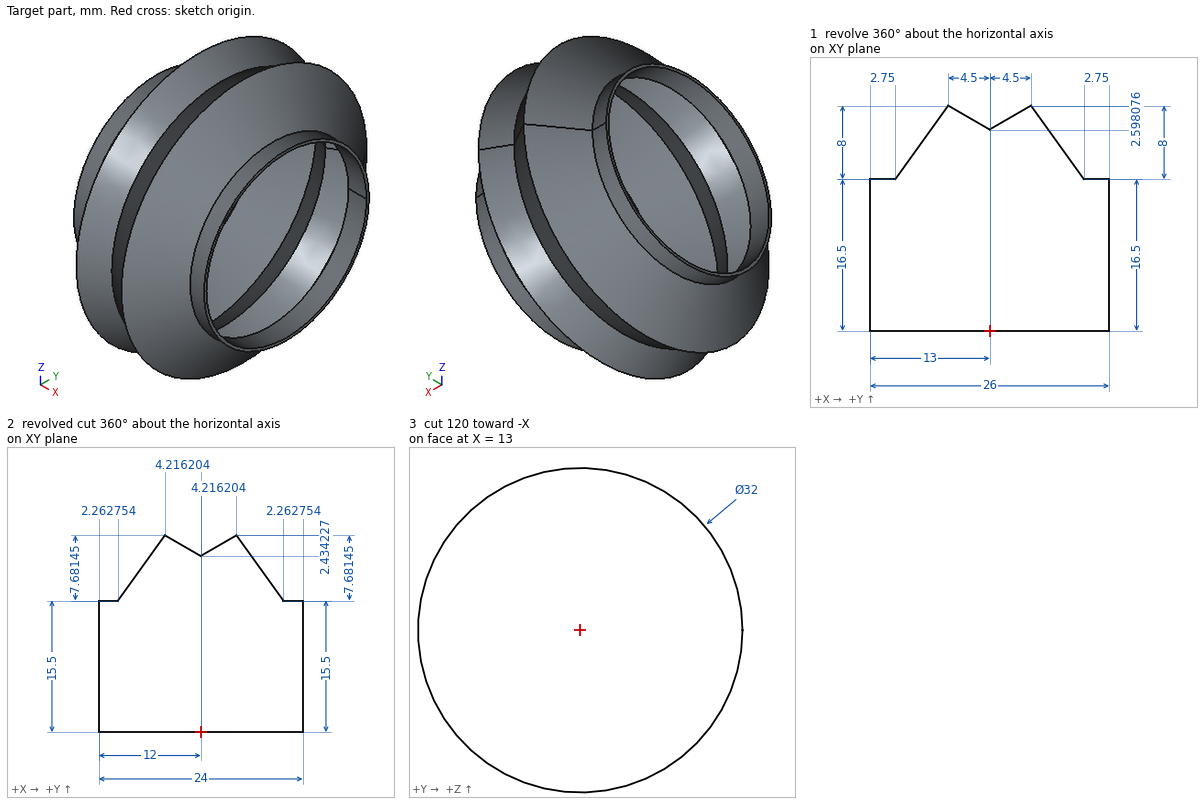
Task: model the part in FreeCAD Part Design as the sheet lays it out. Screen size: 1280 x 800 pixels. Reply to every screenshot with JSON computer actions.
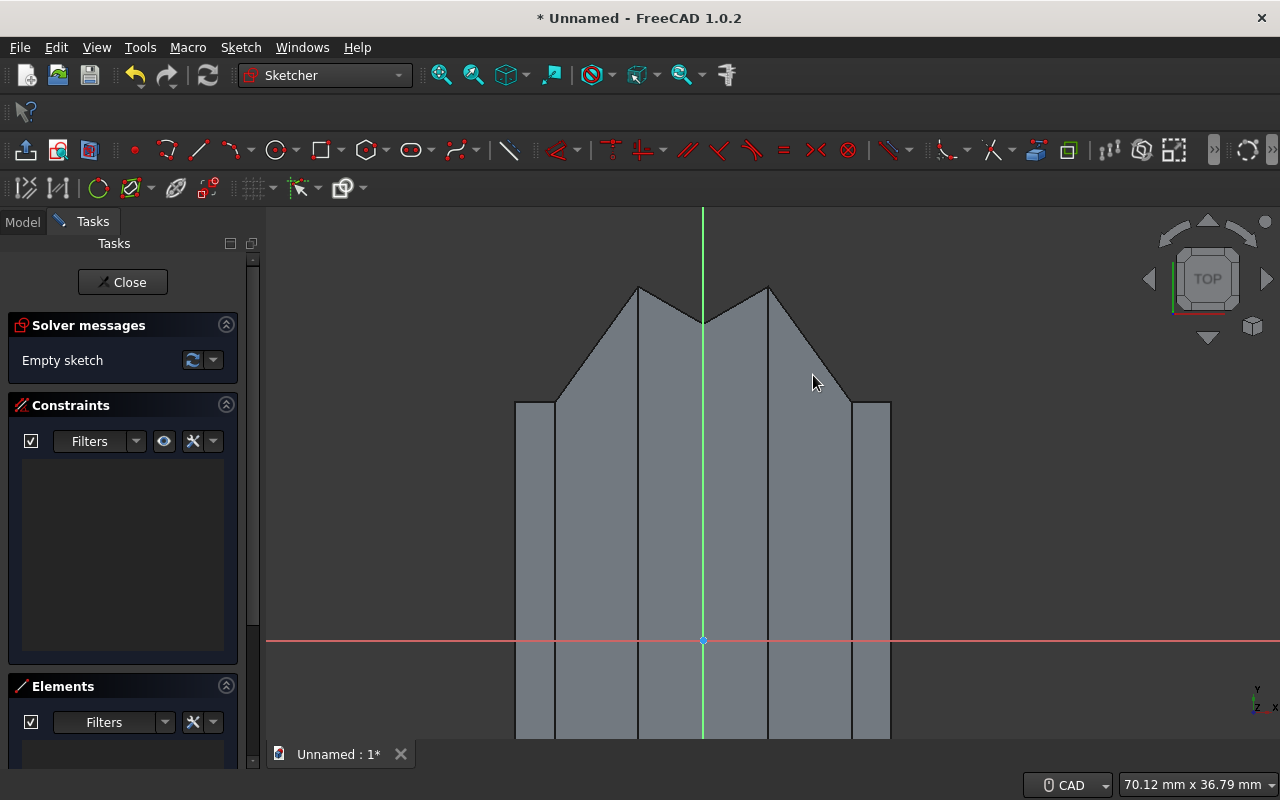
{"action": "left_click", "coordinate": [168, 150]}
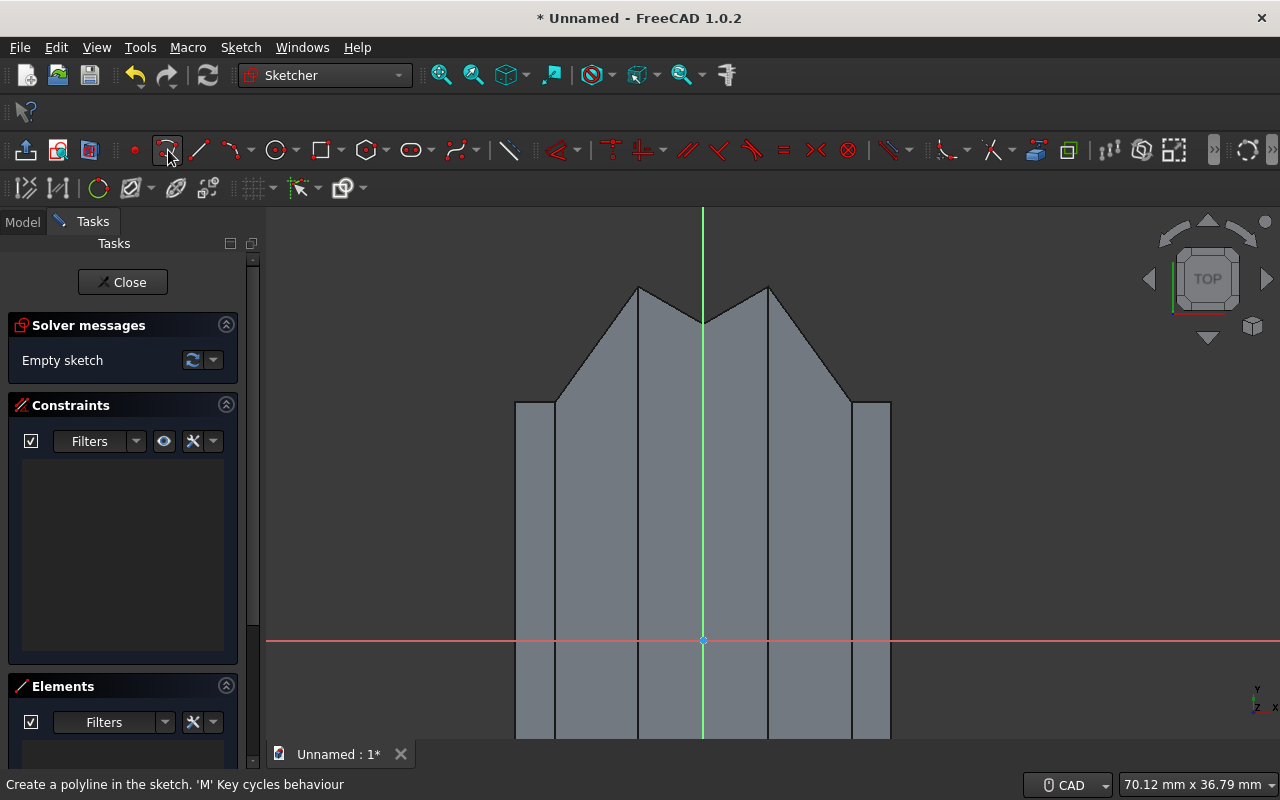
{"action": "left_click", "coordinate": [530, 641]}
{"action": "left_click", "coordinate": [877, 632]}
{"action": "left_click", "coordinate": [877, 417]}
{"action": "left_click", "coordinate": [844, 417]}
{"action": "left_click", "coordinate": [764, 306]}
{"action": "left_click", "coordinate": [703, 341]}
{"action": "left_click", "coordinate": [642, 306]}
{"action": "left_click", "coordinate": [563, 417]}
{"action": "left_click", "coordinate": [530, 417]}
{"action": "left_click", "coordinate": [530, 641]}
{"action": "key", "text": "Escape"}
{"action": "key", "text": "Escape"}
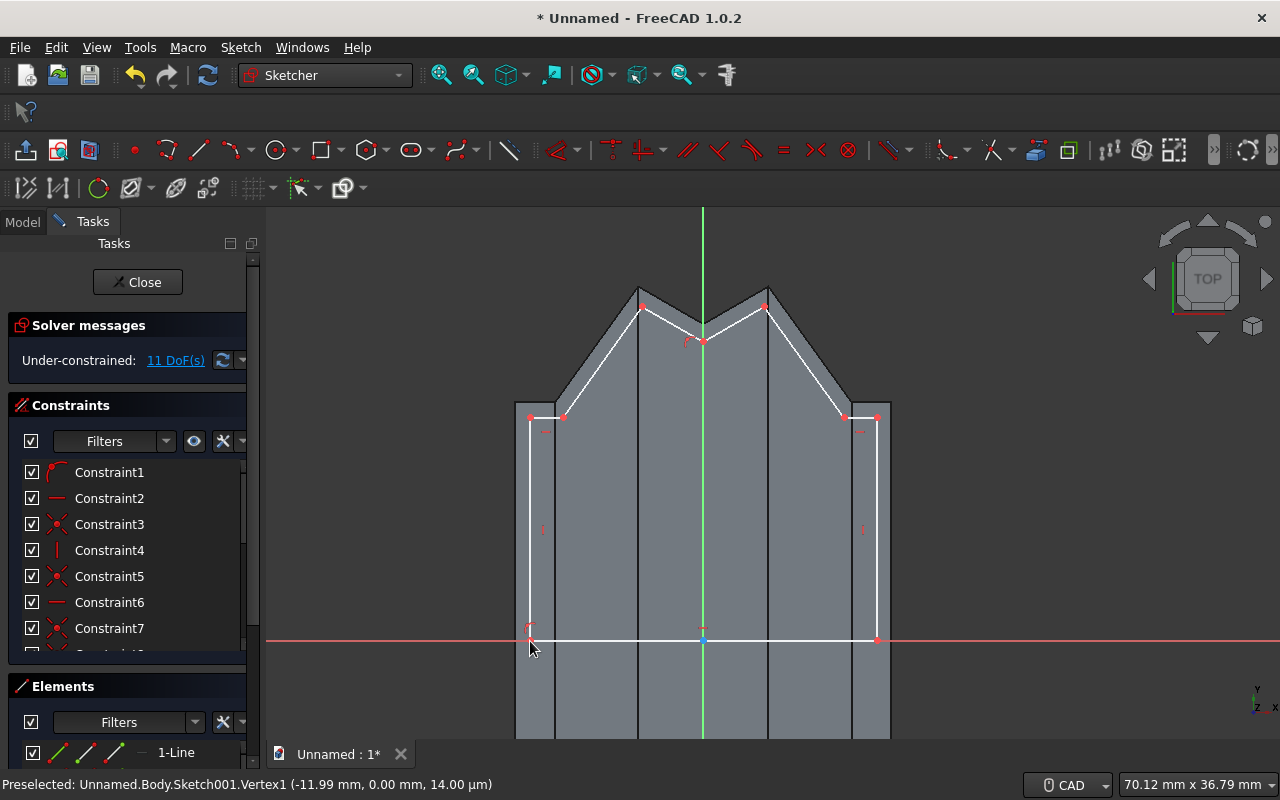
{"action": "key", "text": "d"}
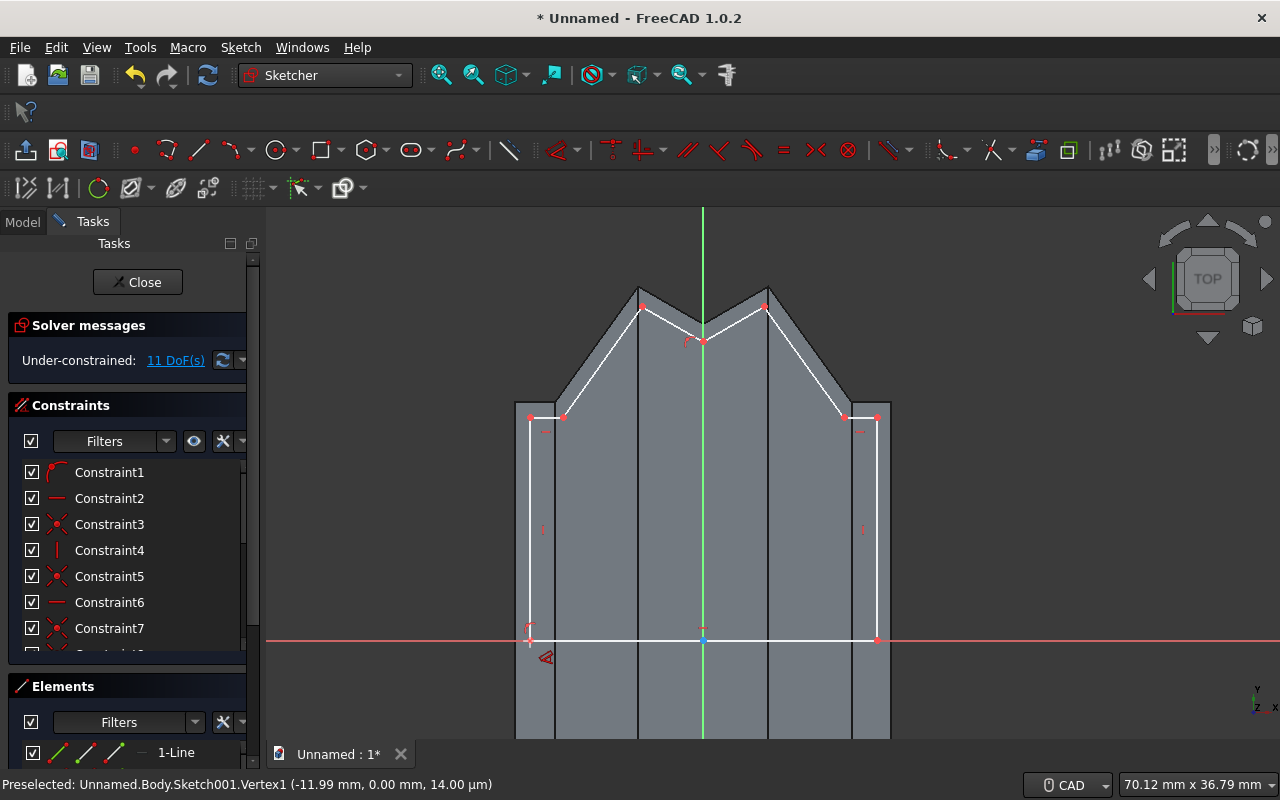
{"action": "left_click", "coordinate": [634, 641]}
{"action": "left_click", "coordinate": [624, 675]}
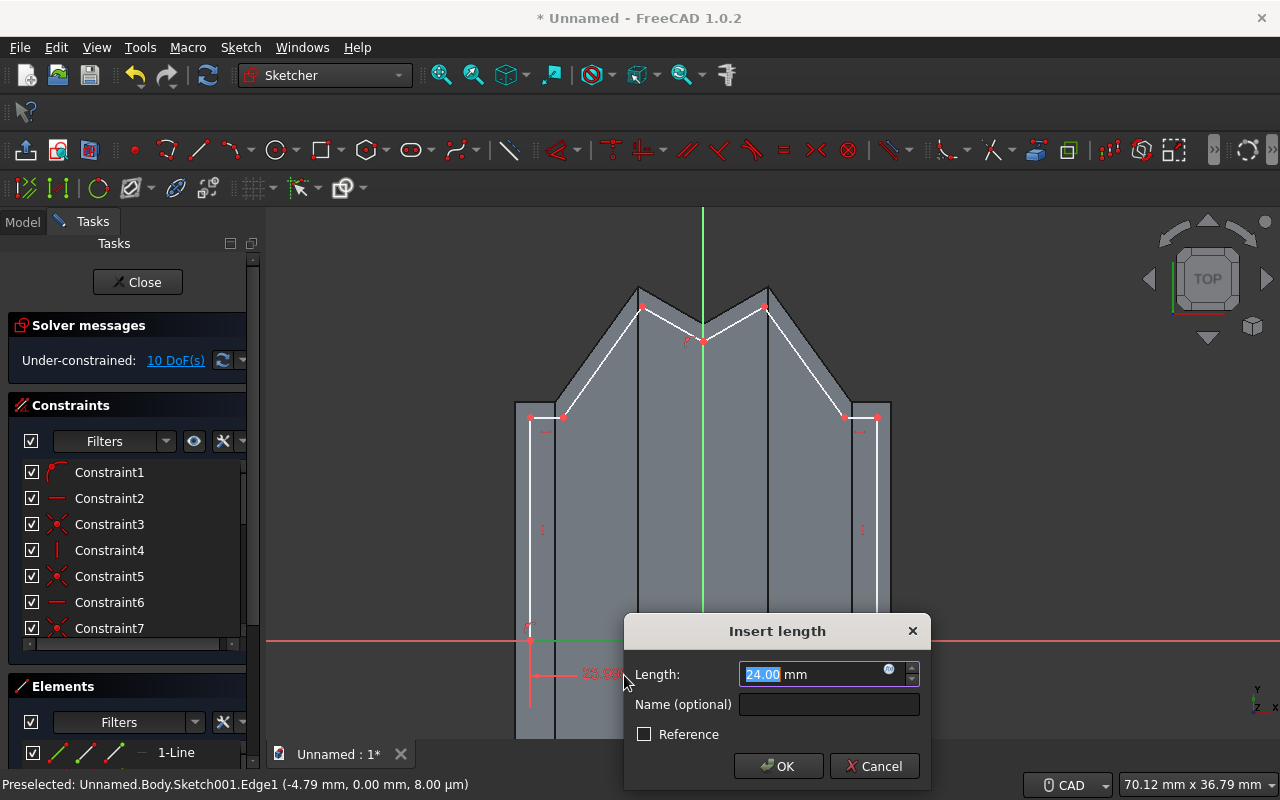
{"action": "type", "text": "24"}
{"action": "key", "text": "Return"}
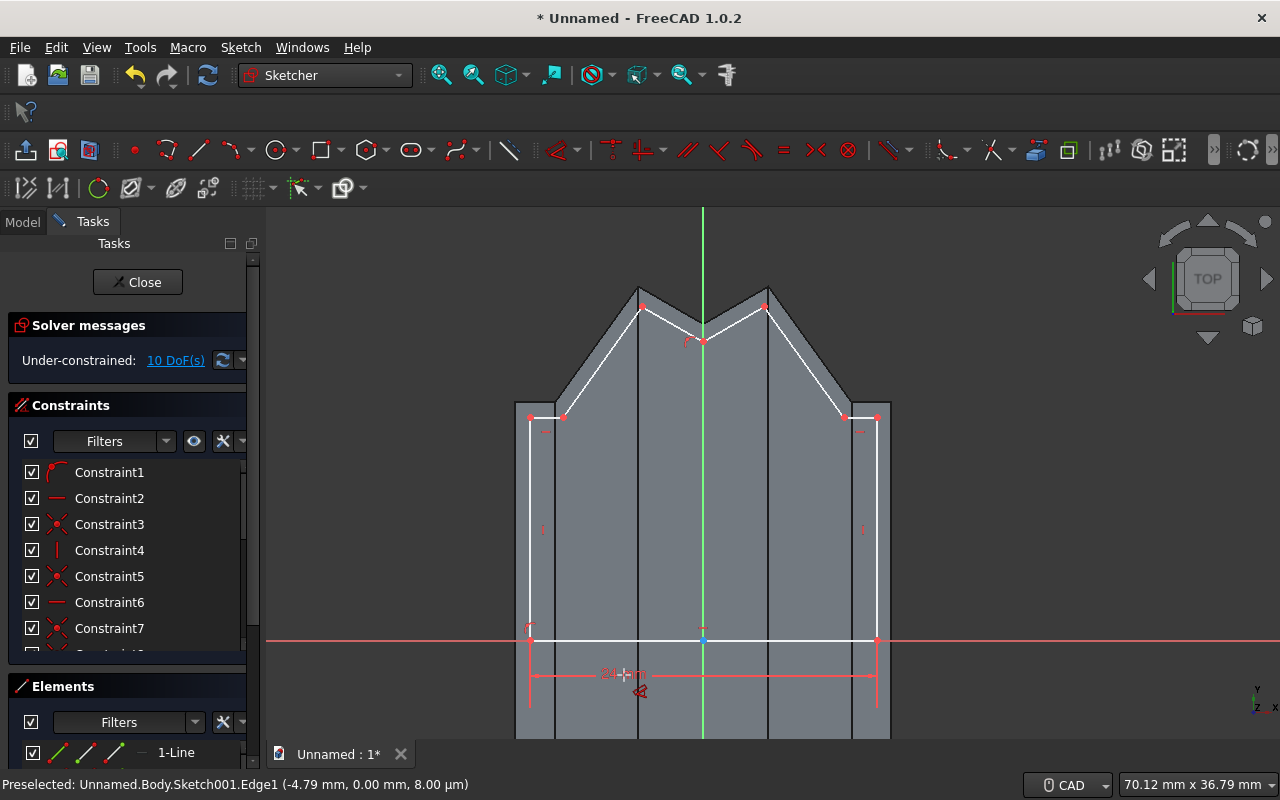
{"action": "left_click", "coordinate": [530, 641]}
{"action": "left_click", "coordinate": [617, 607]}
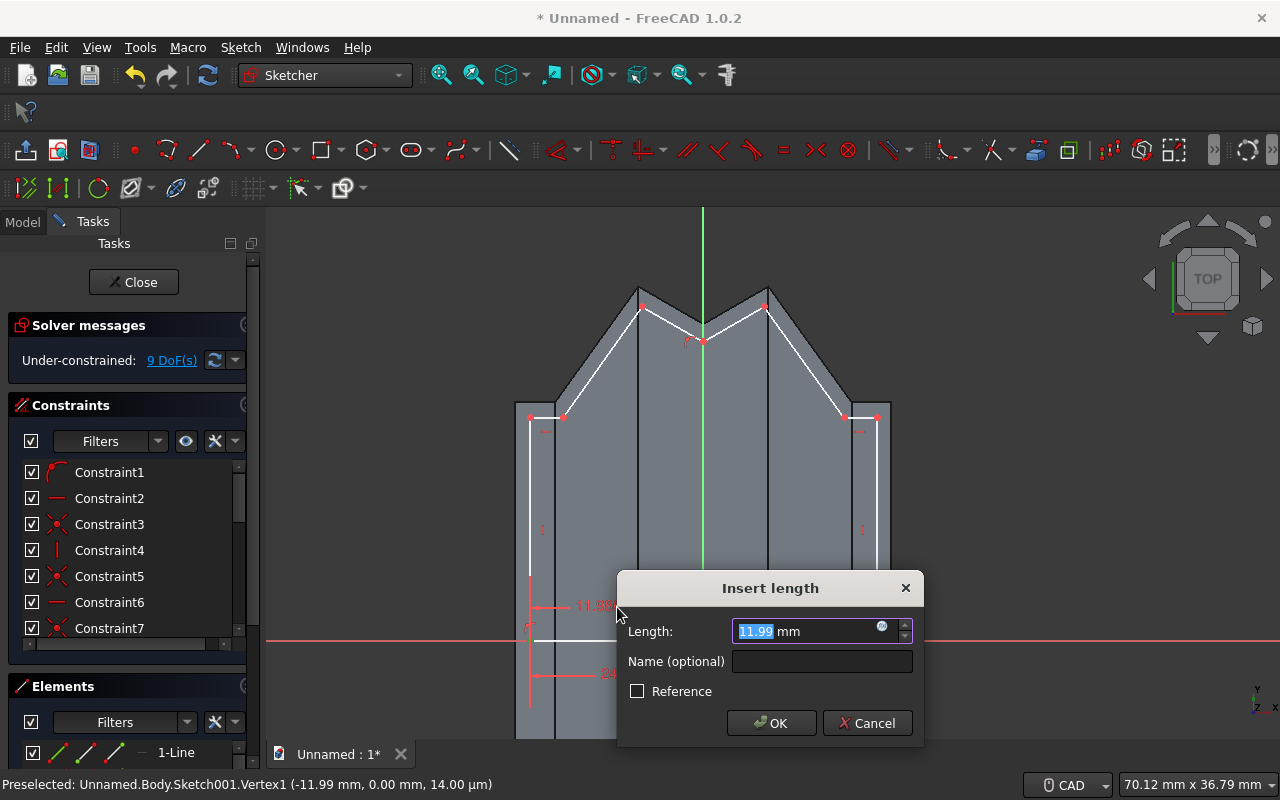
{"action": "type", "text": "12"}
{"action": "key", "text": "Return"}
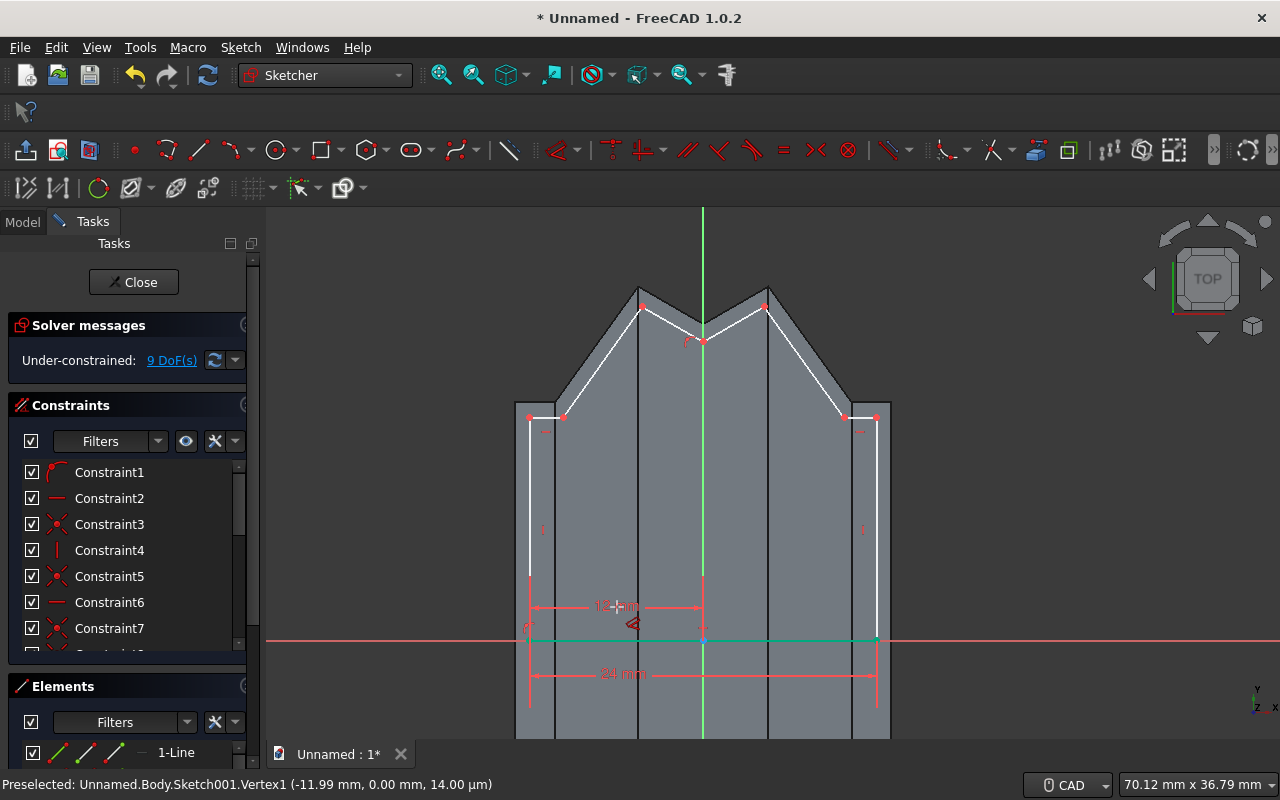
{"action": "left_click", "coordinate": [877, 574]}
{"action": "left_click", "coordinate": [911, 529]}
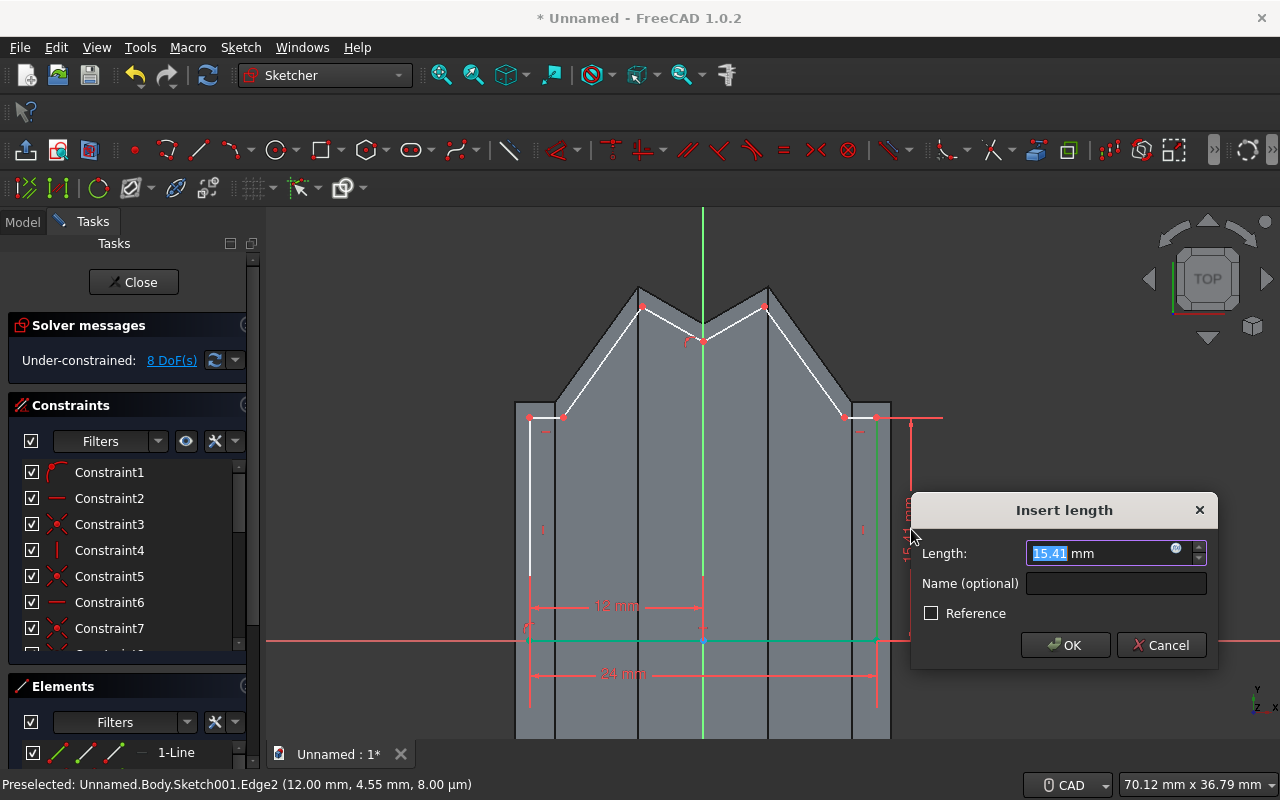
{"action": "type", "text": "15.5"}
{"action": "key", "text": "Return"}